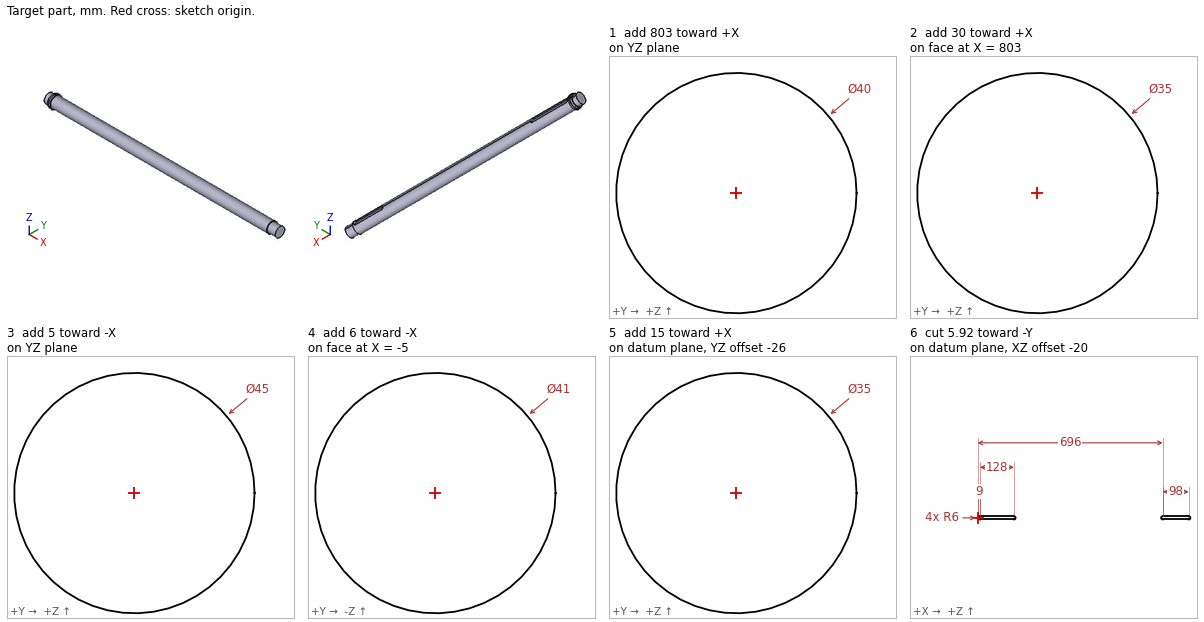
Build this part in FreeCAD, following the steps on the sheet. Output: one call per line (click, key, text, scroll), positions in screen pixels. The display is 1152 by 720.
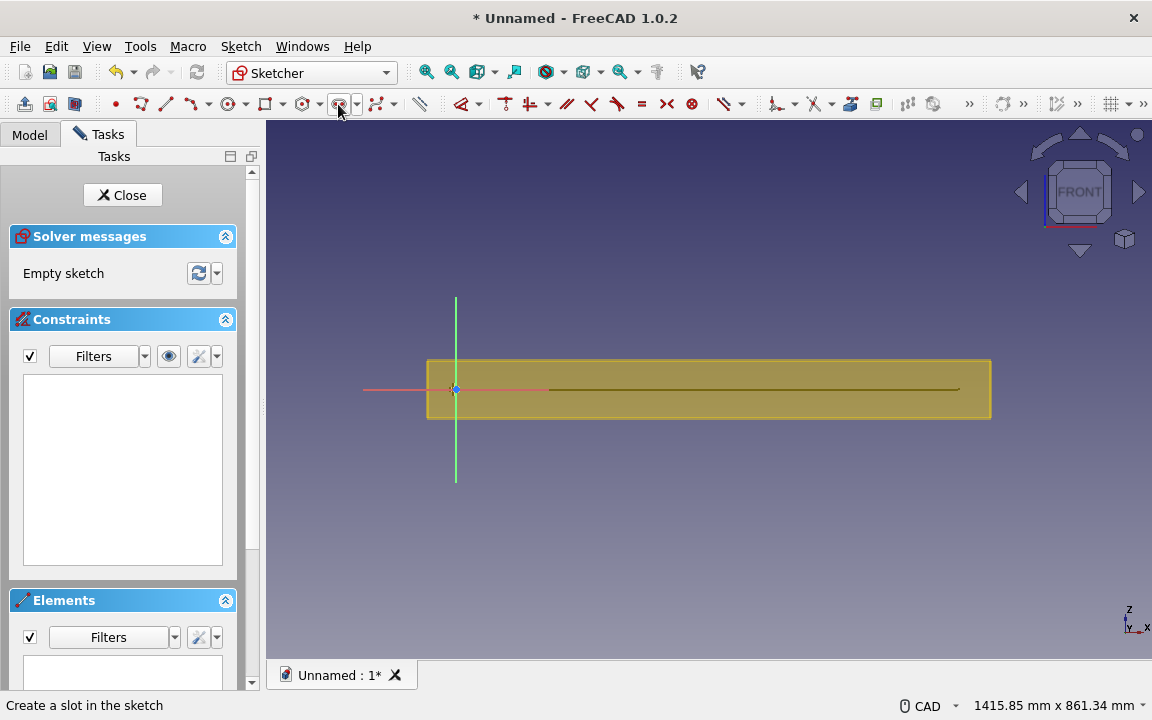
scroll(462, 390, up, 9)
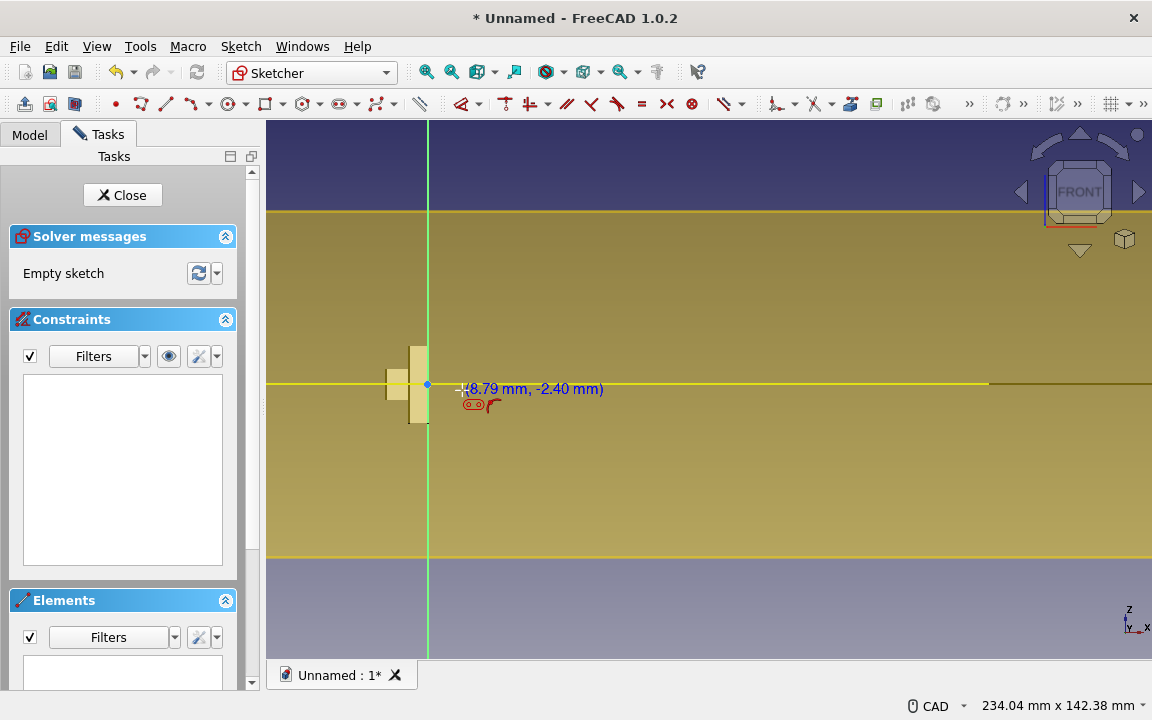
click(462, 384)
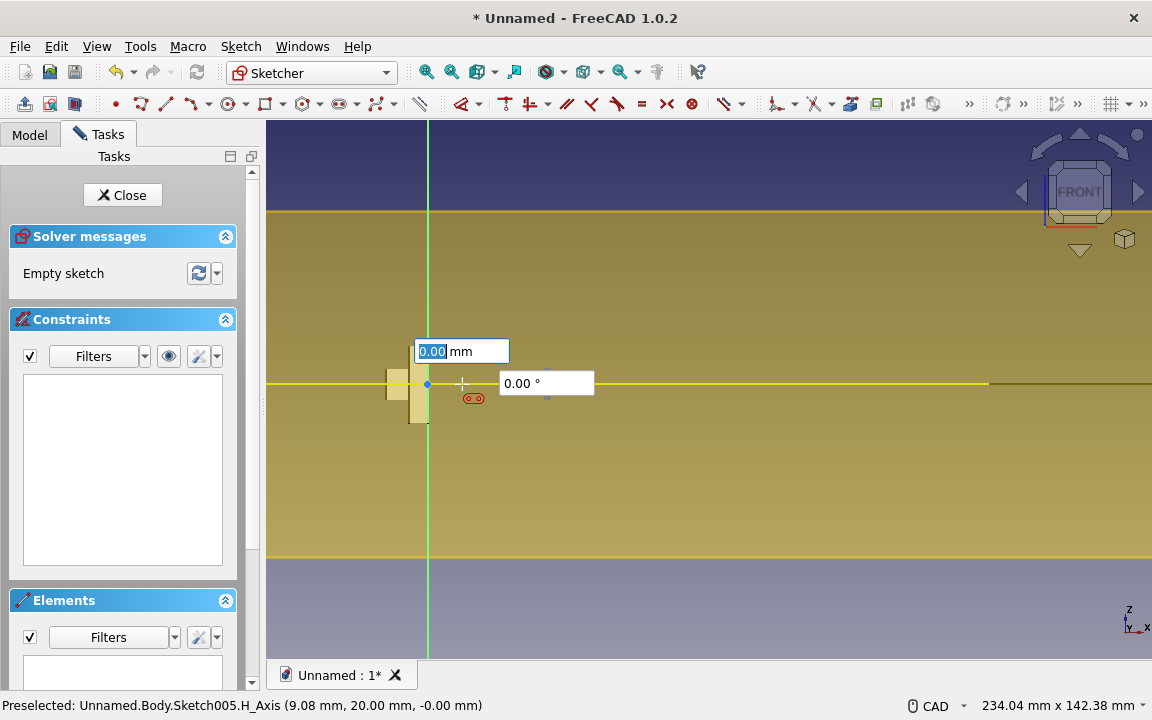
scroll(383, 391, down, 9)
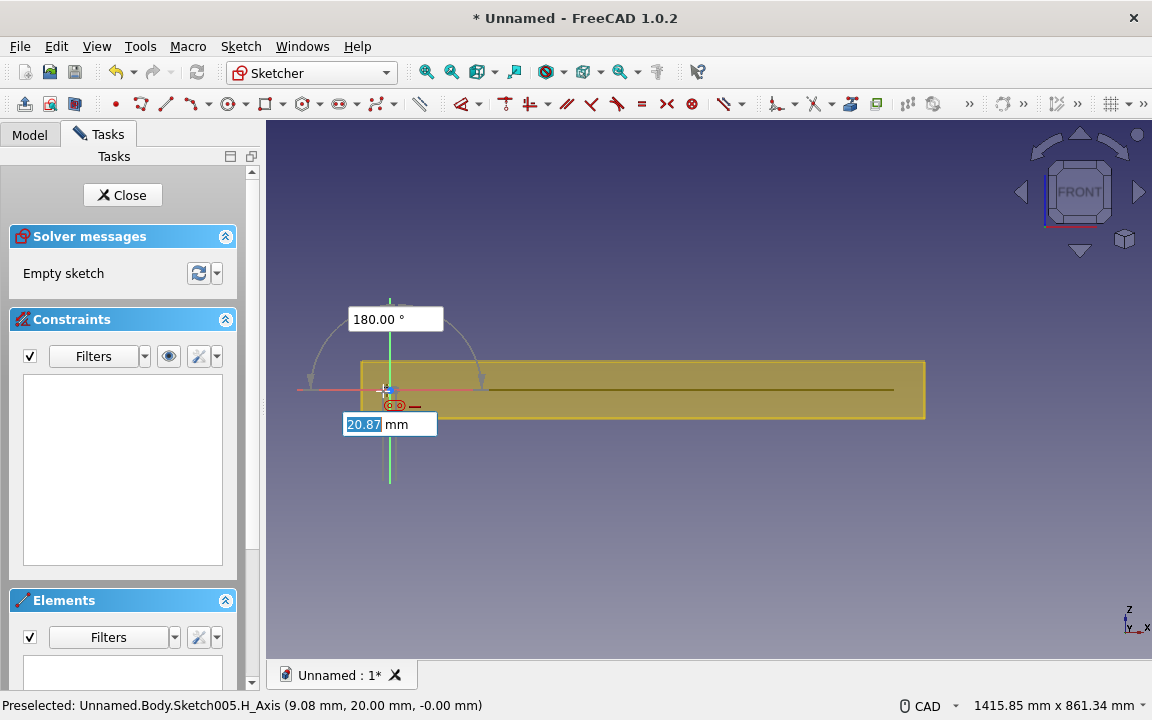
click(476, 381)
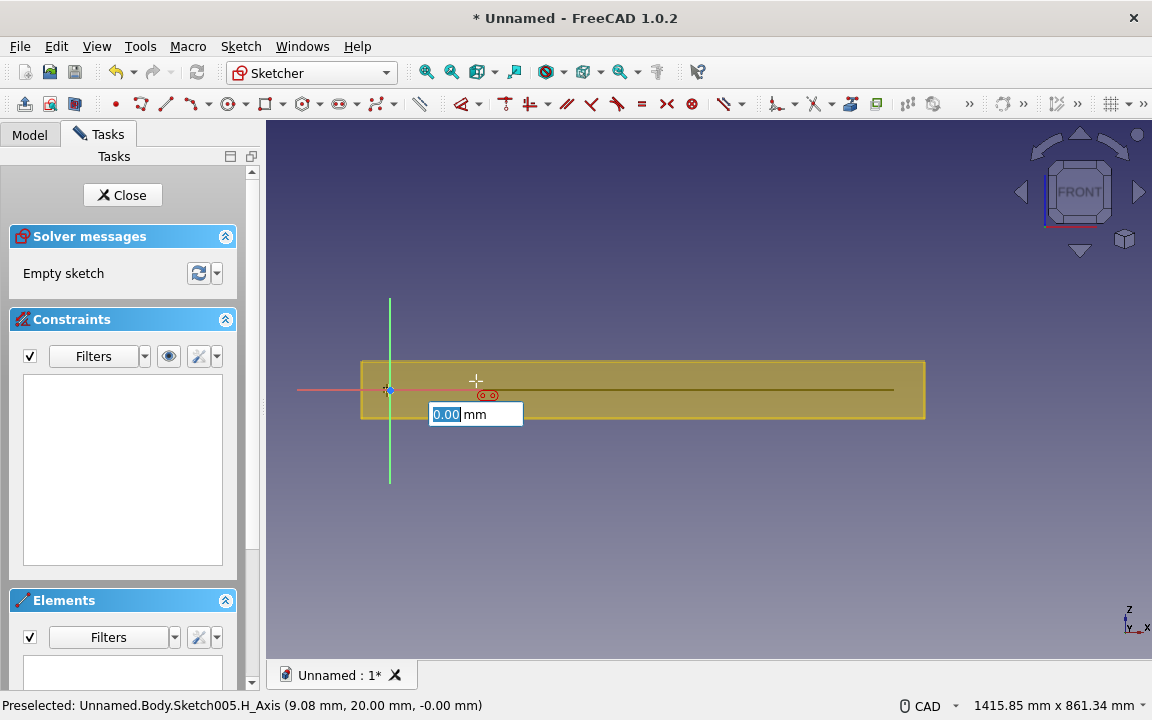
scroll(436, 394, up, 8)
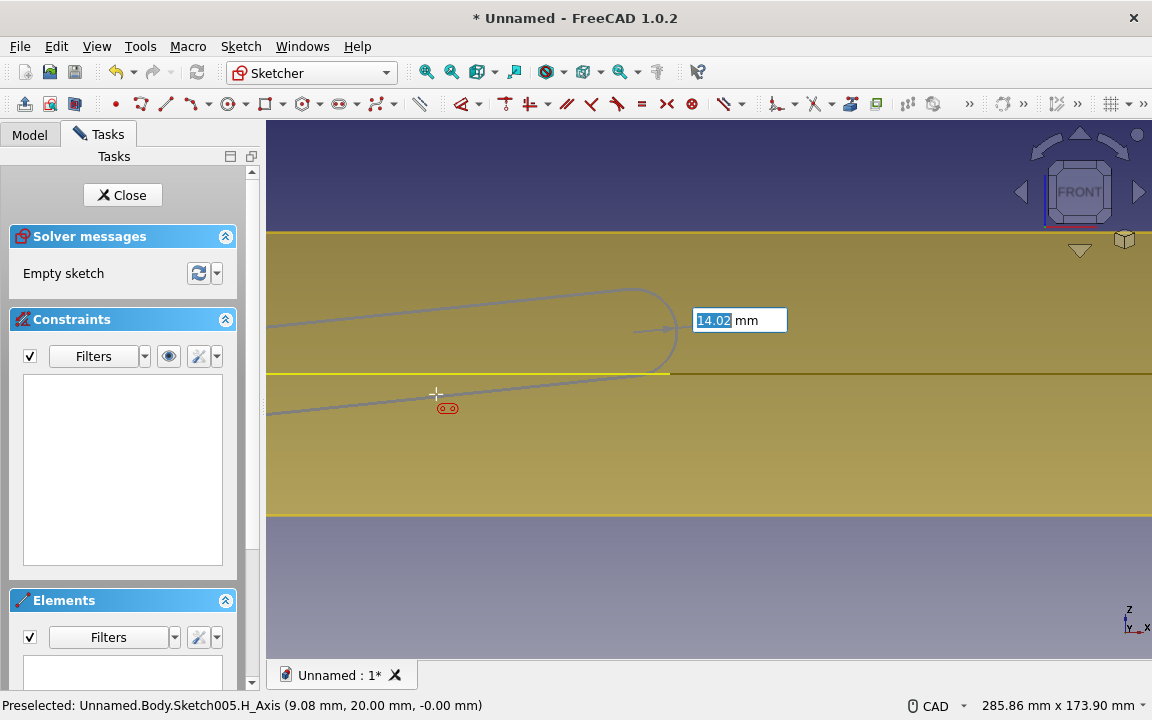
click(436, 392)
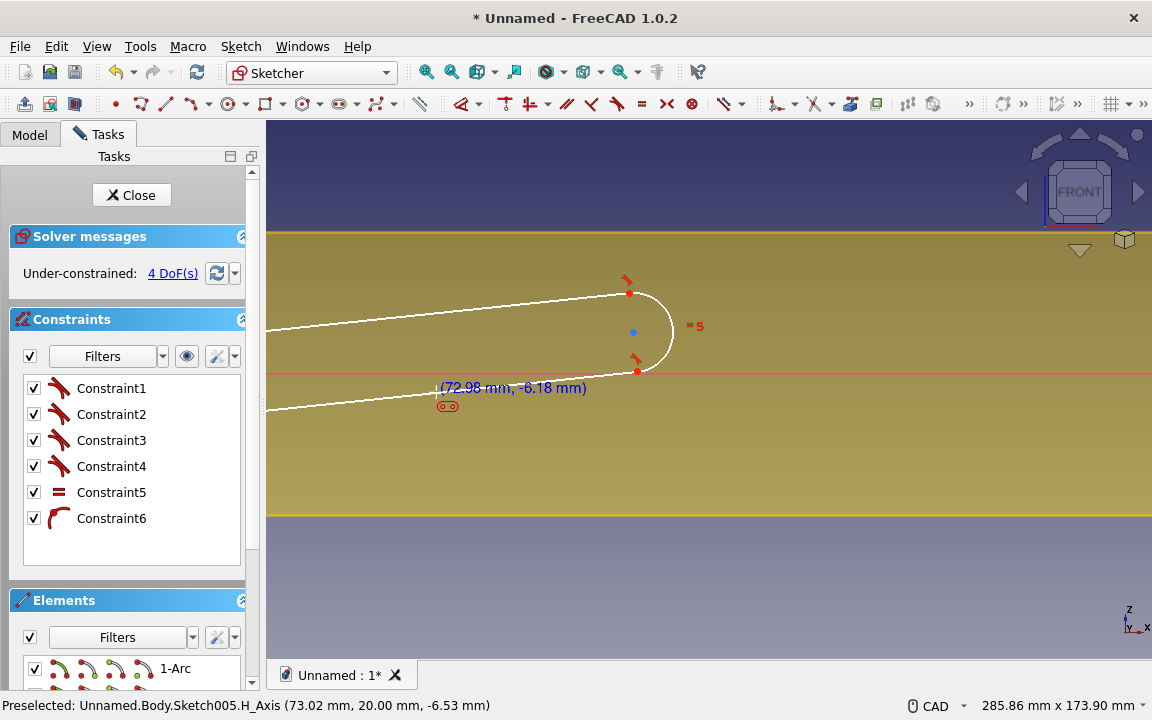
scroll(436, 393, down, 8)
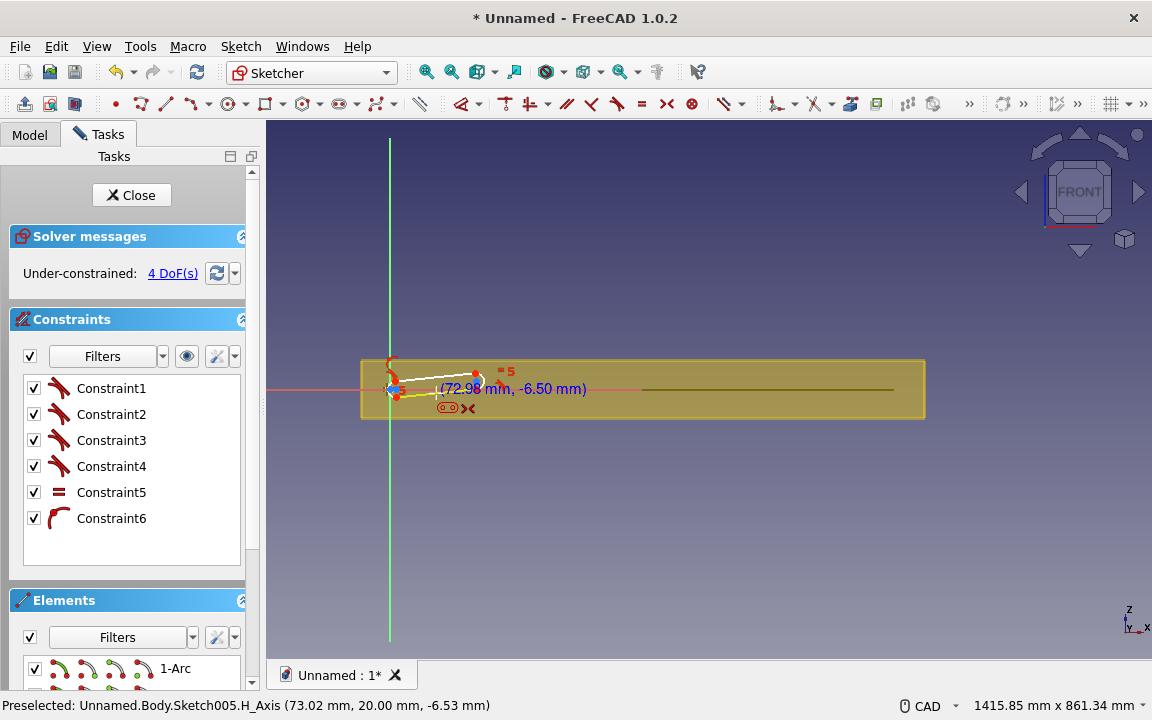
scroll(826, 390, up, 9)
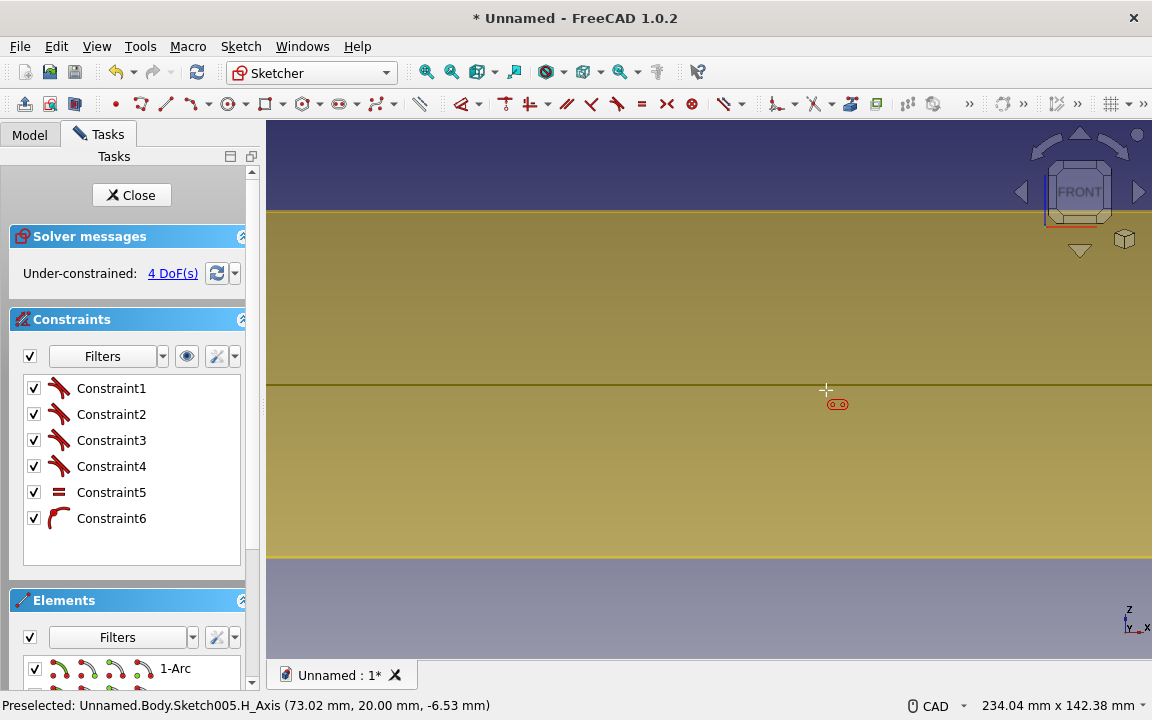
scroll(826, 390, down, 9)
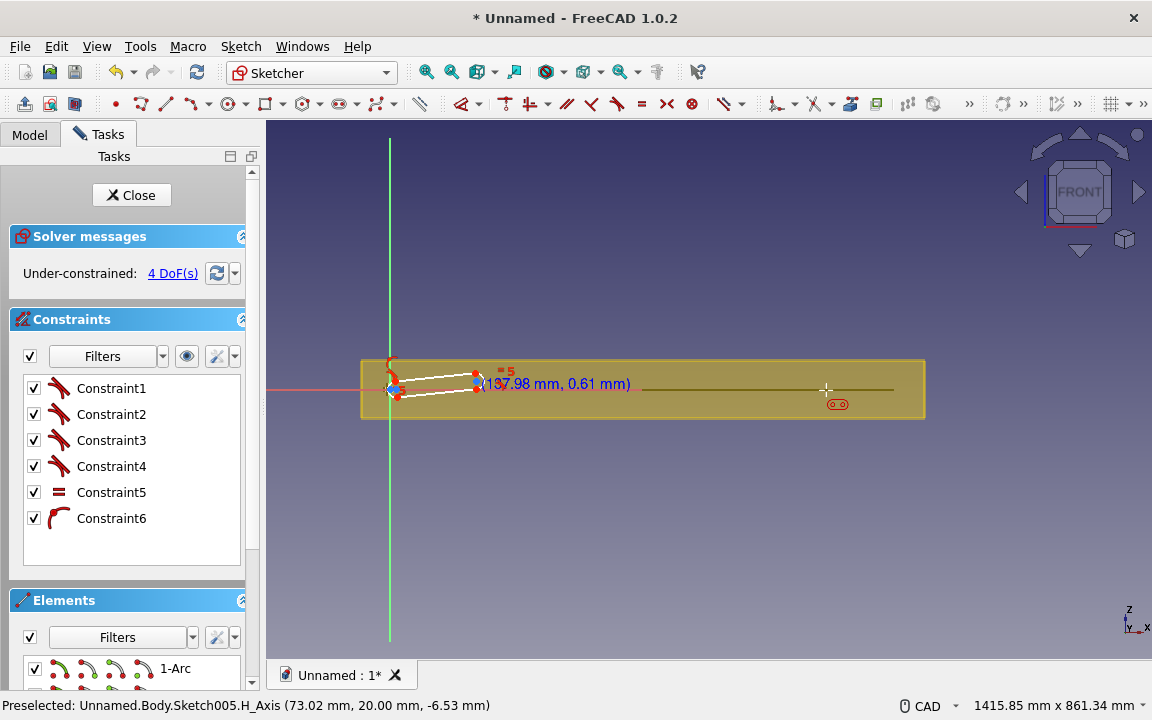
click(826, 390)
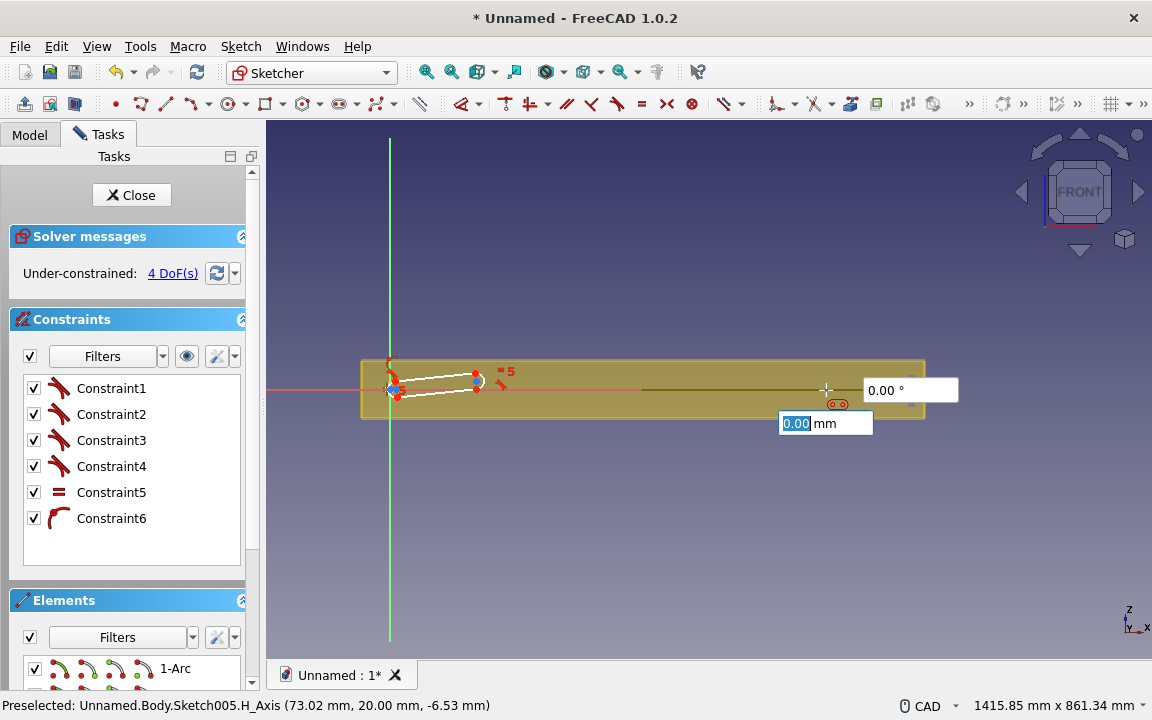
click(887, 381)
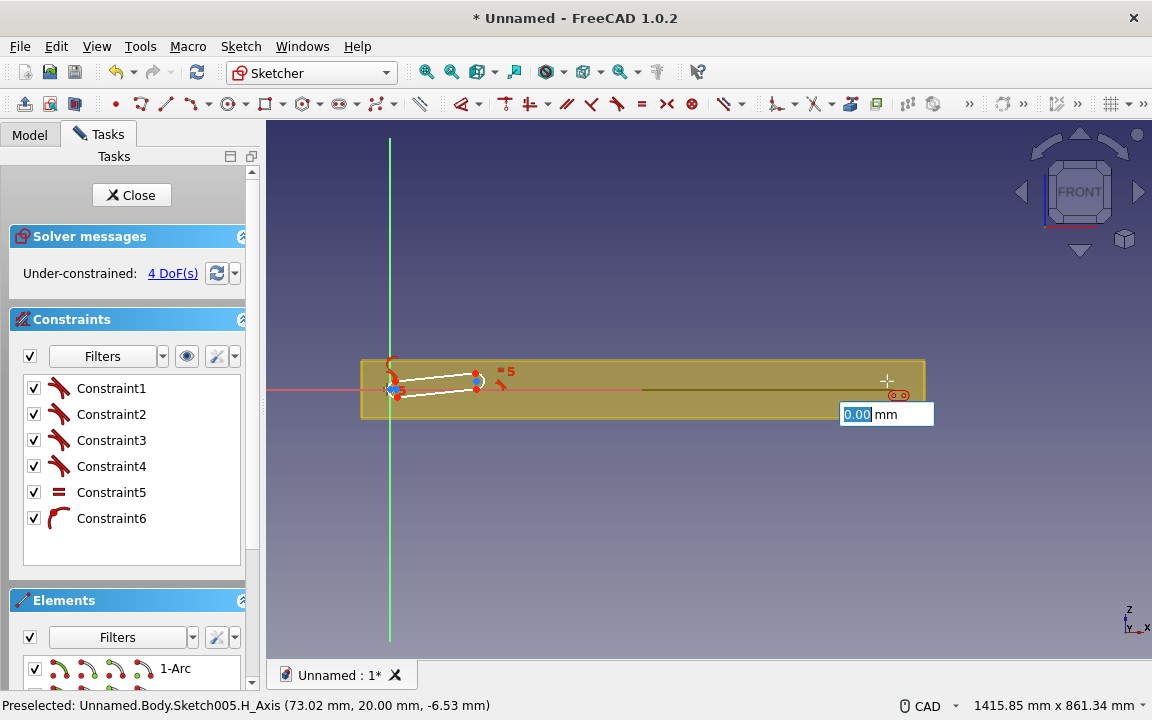
scroll(857, 386, up, 8)